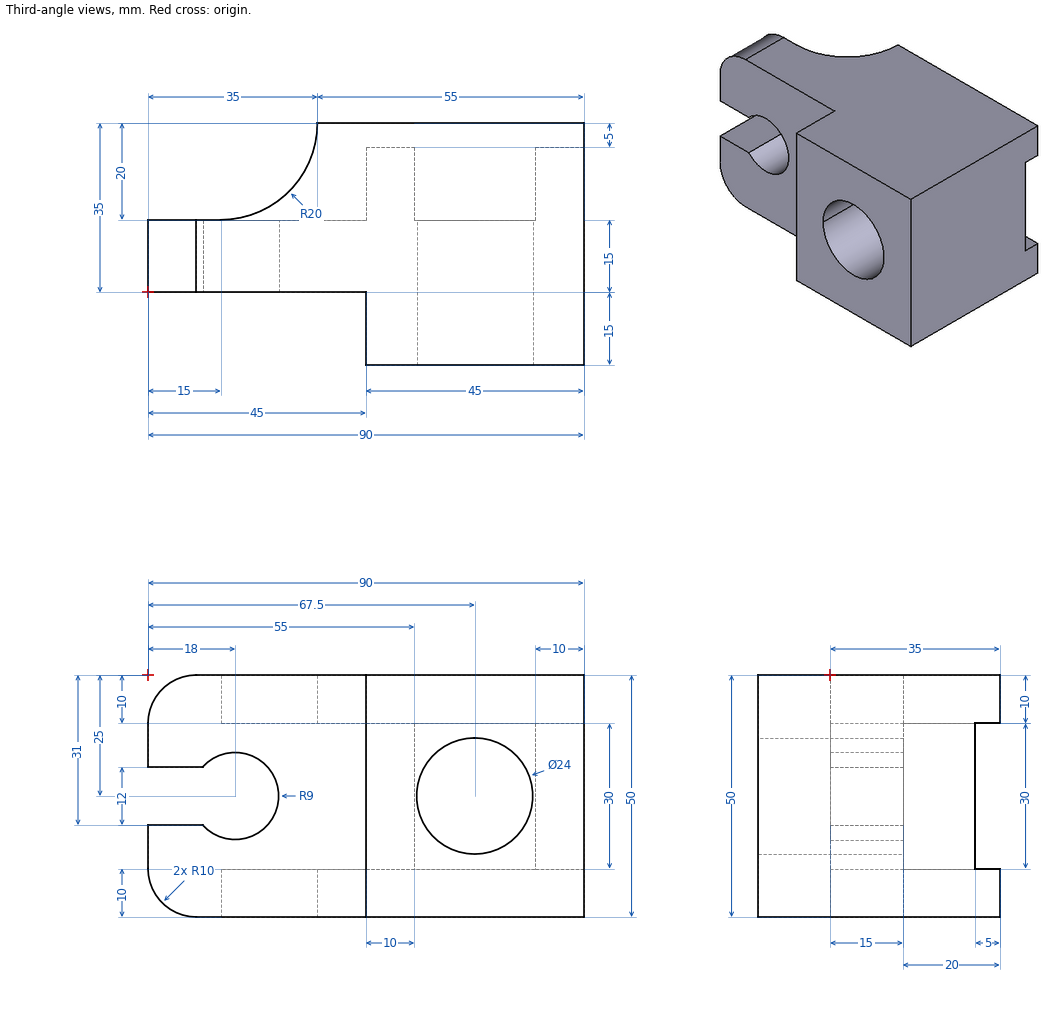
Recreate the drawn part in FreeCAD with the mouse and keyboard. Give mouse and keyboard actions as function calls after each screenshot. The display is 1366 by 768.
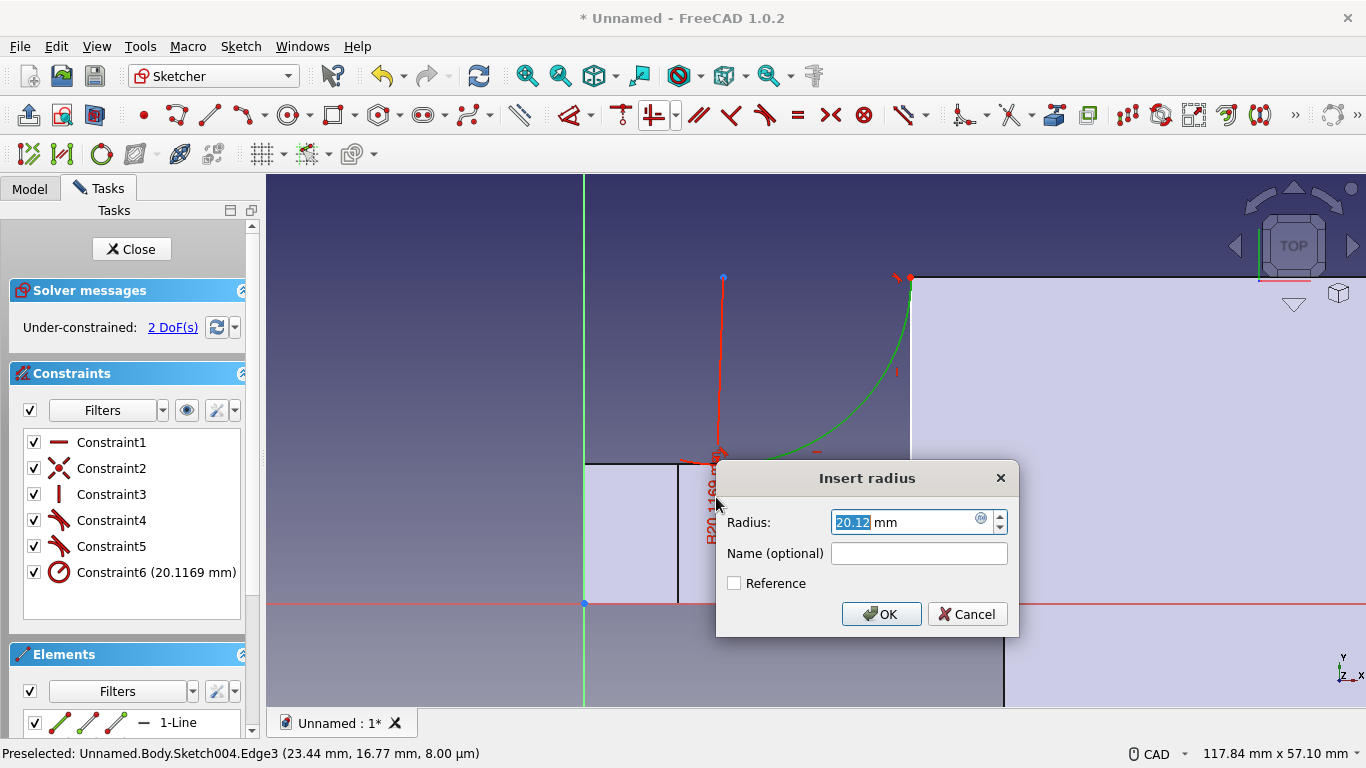
text(20)
key(Return)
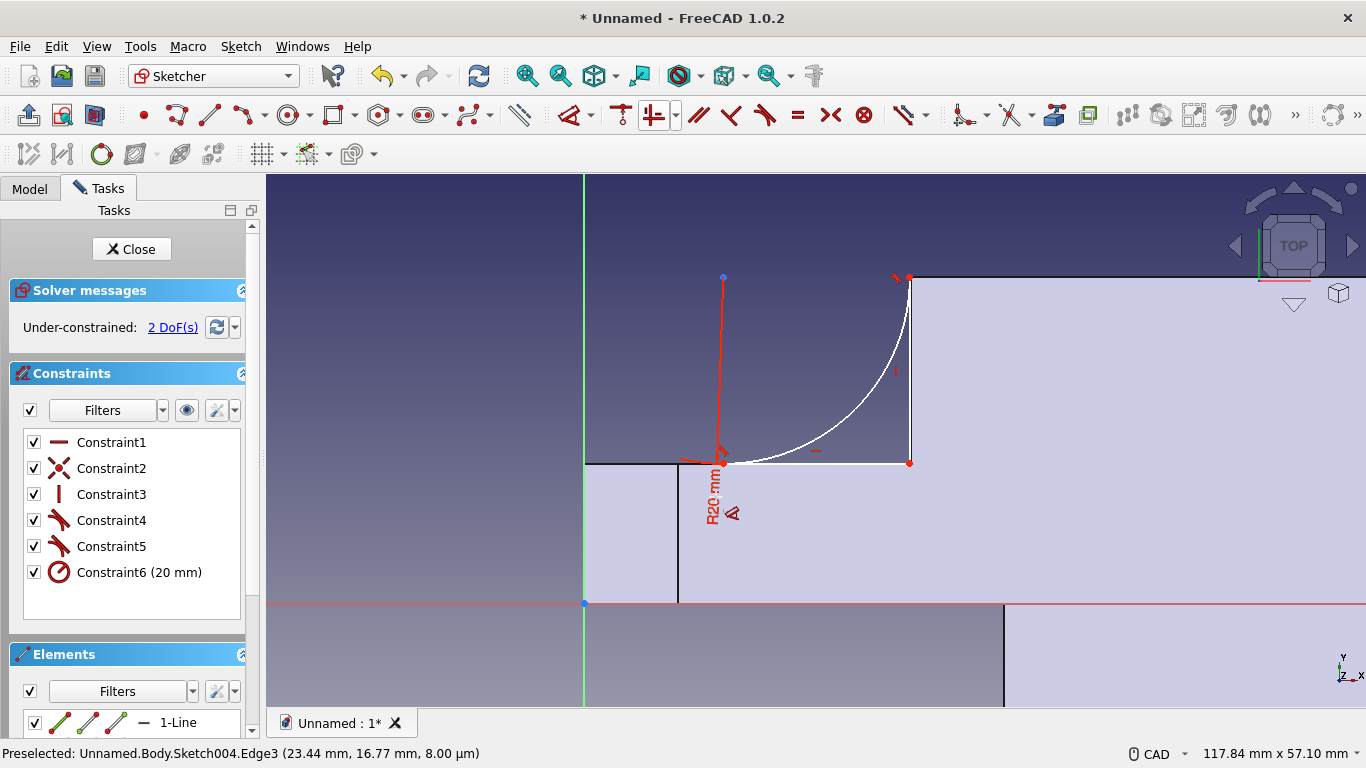
click(723, 464)
click(654, 638)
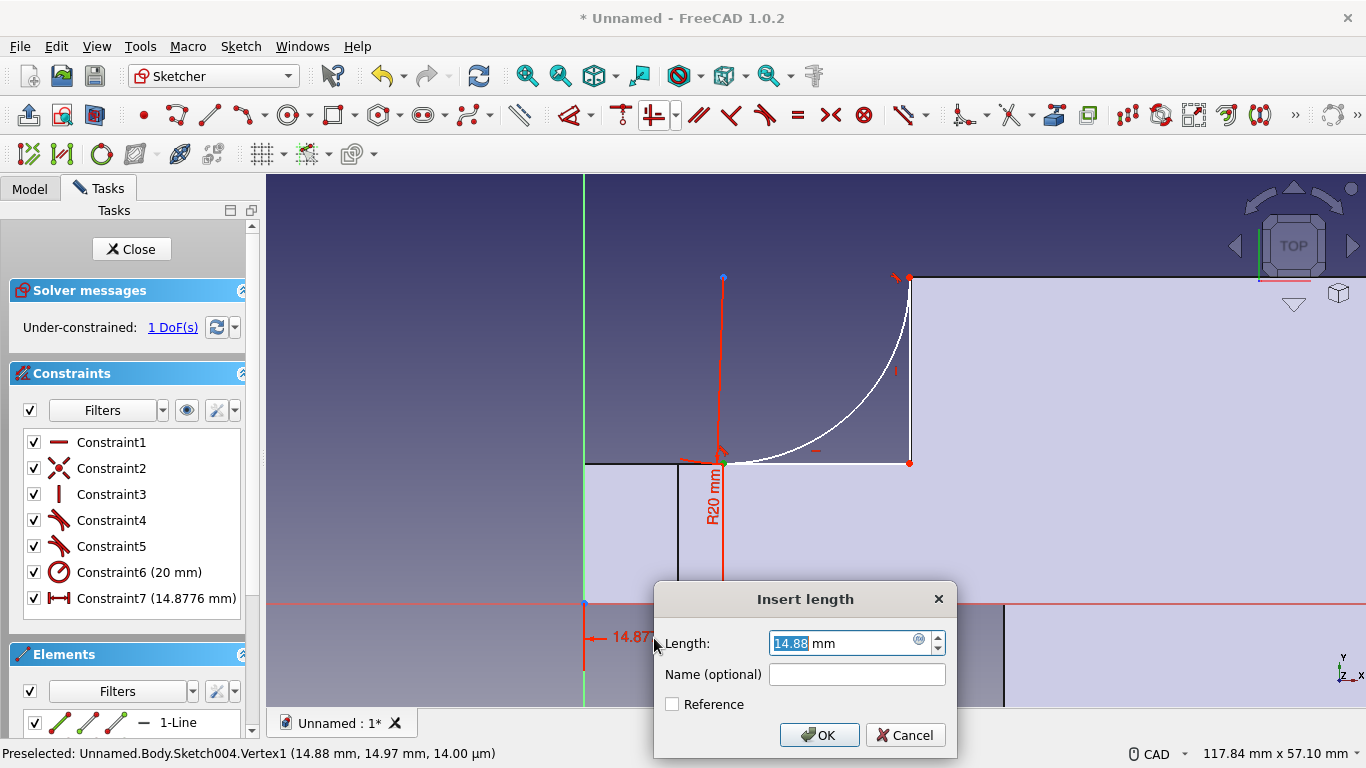
text(15)
key(Return)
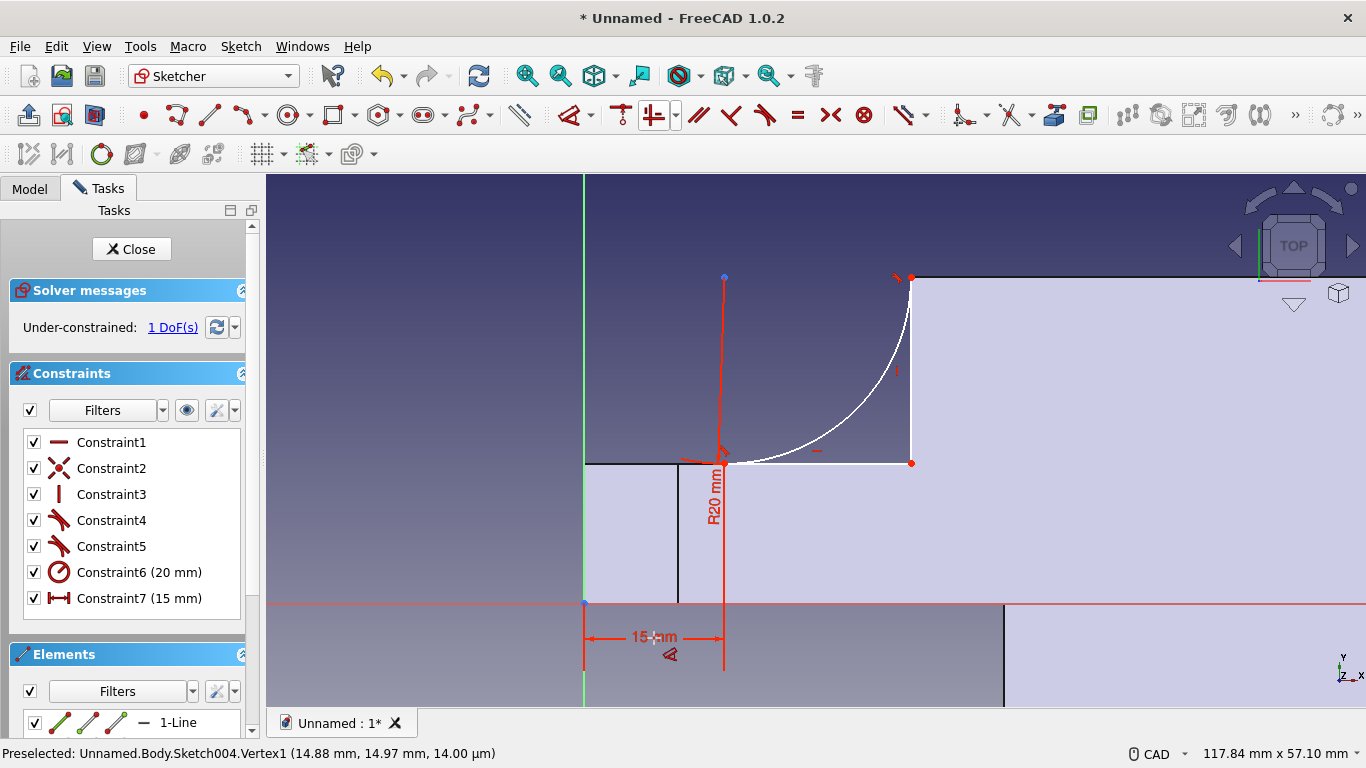
click(724, 464)
click(550, 534)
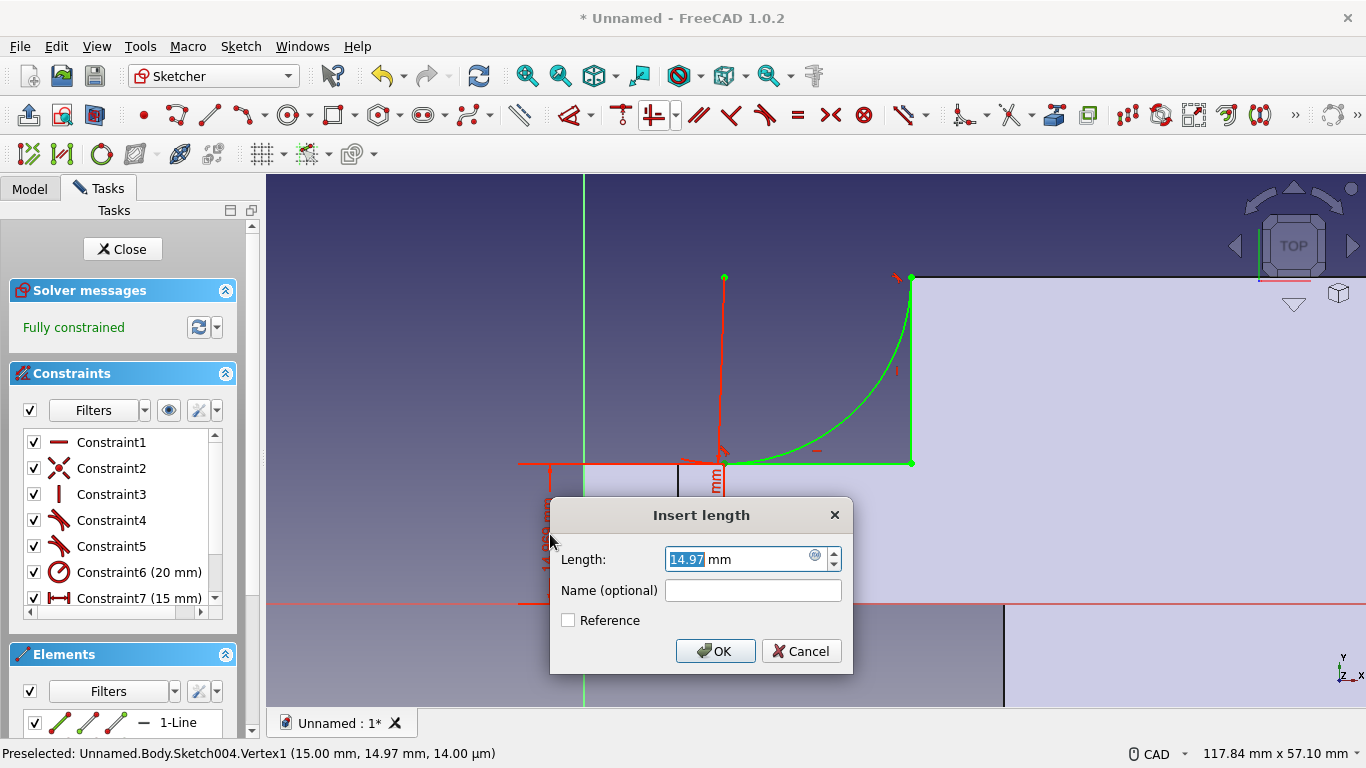
text(15)
key(Return)
key(Escape)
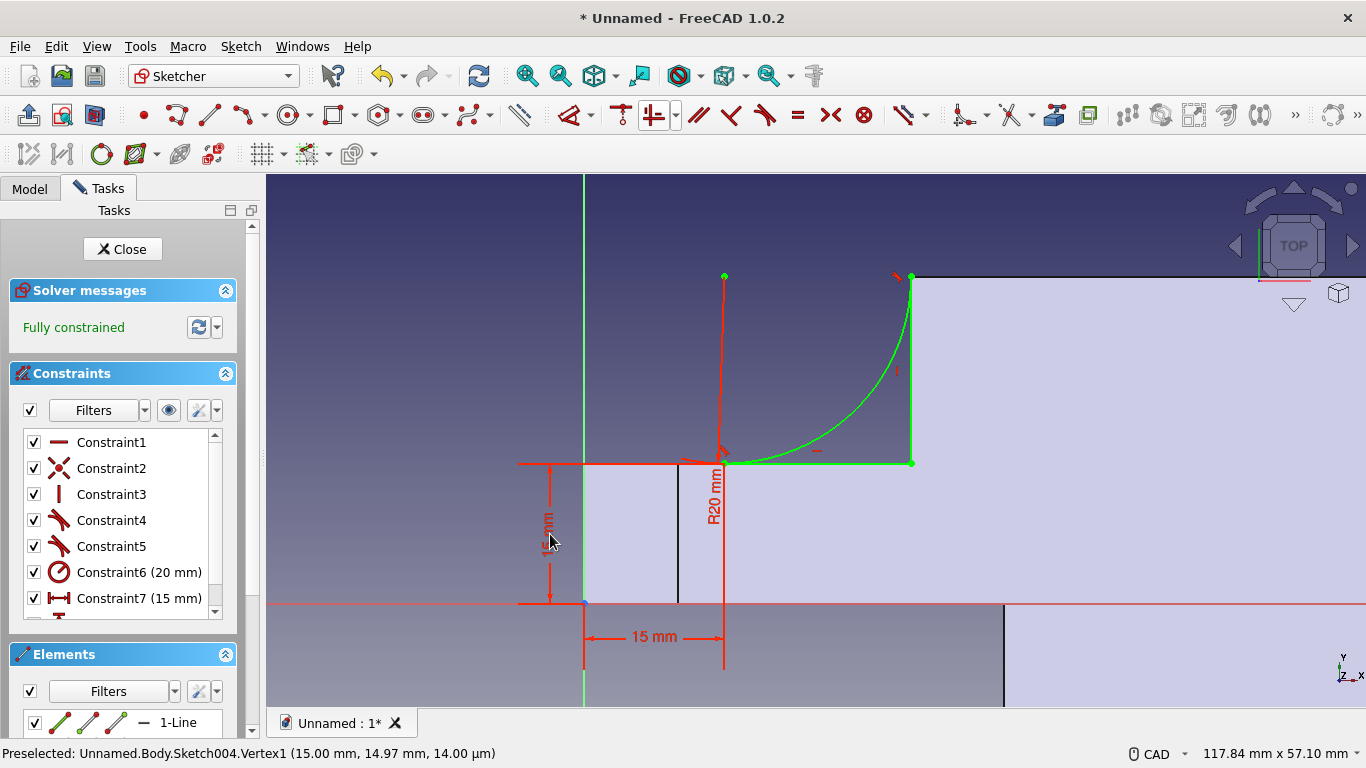
click(123, 249)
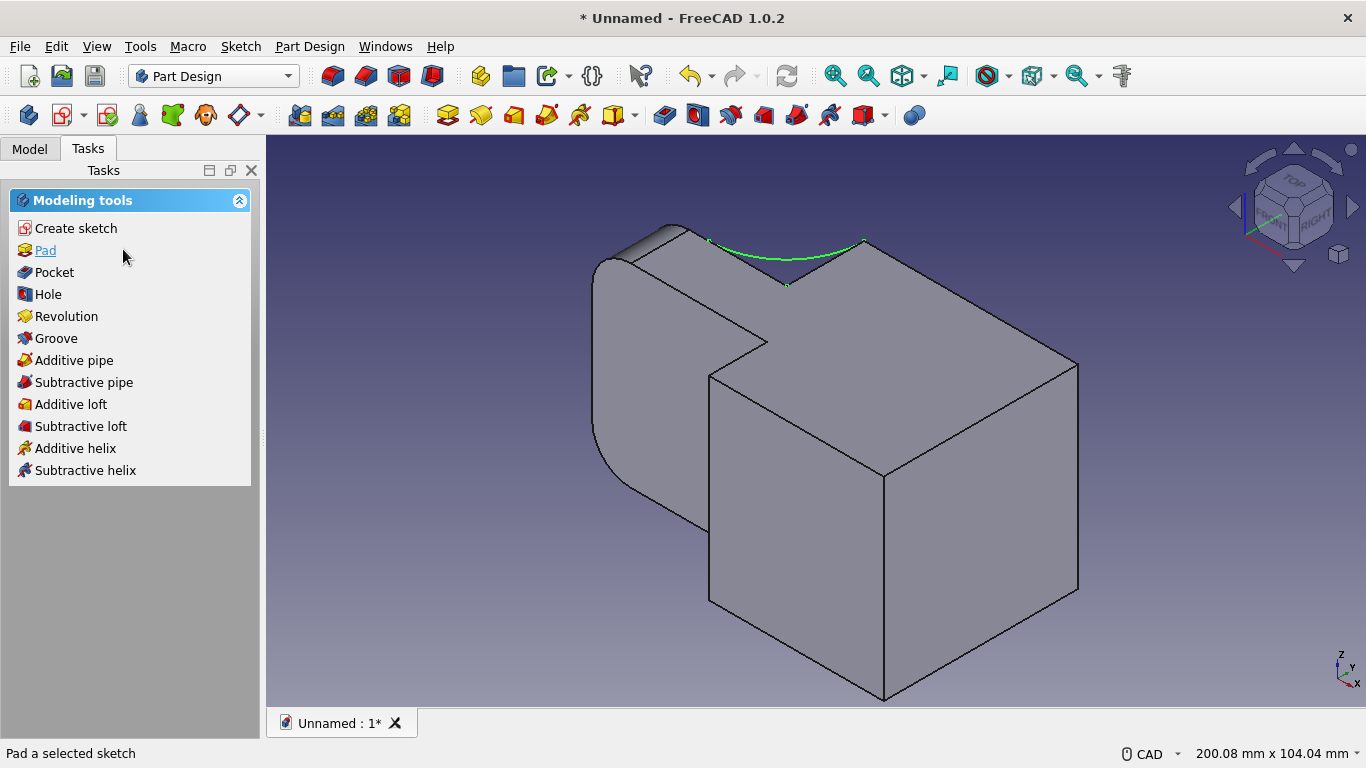
click(448, 116)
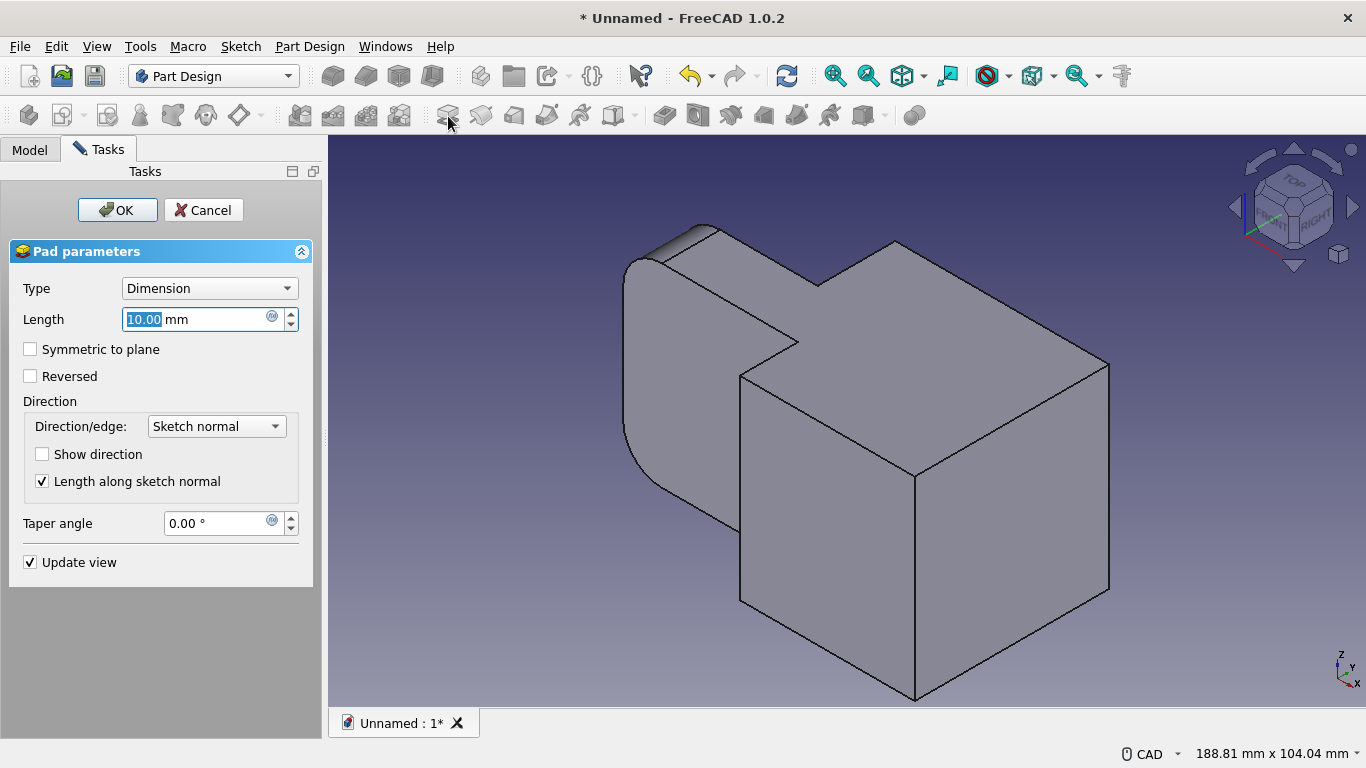
text(10)
key(Tab)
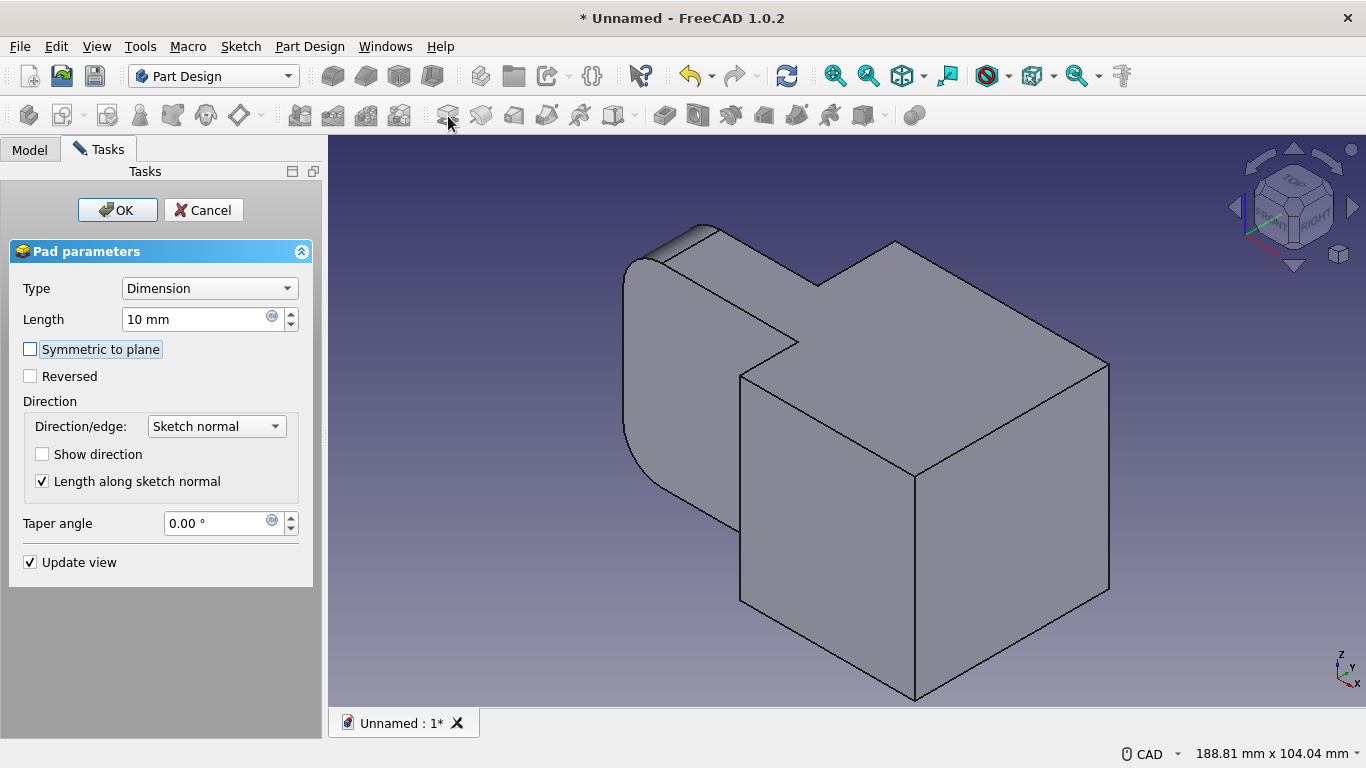
click(31, 376)